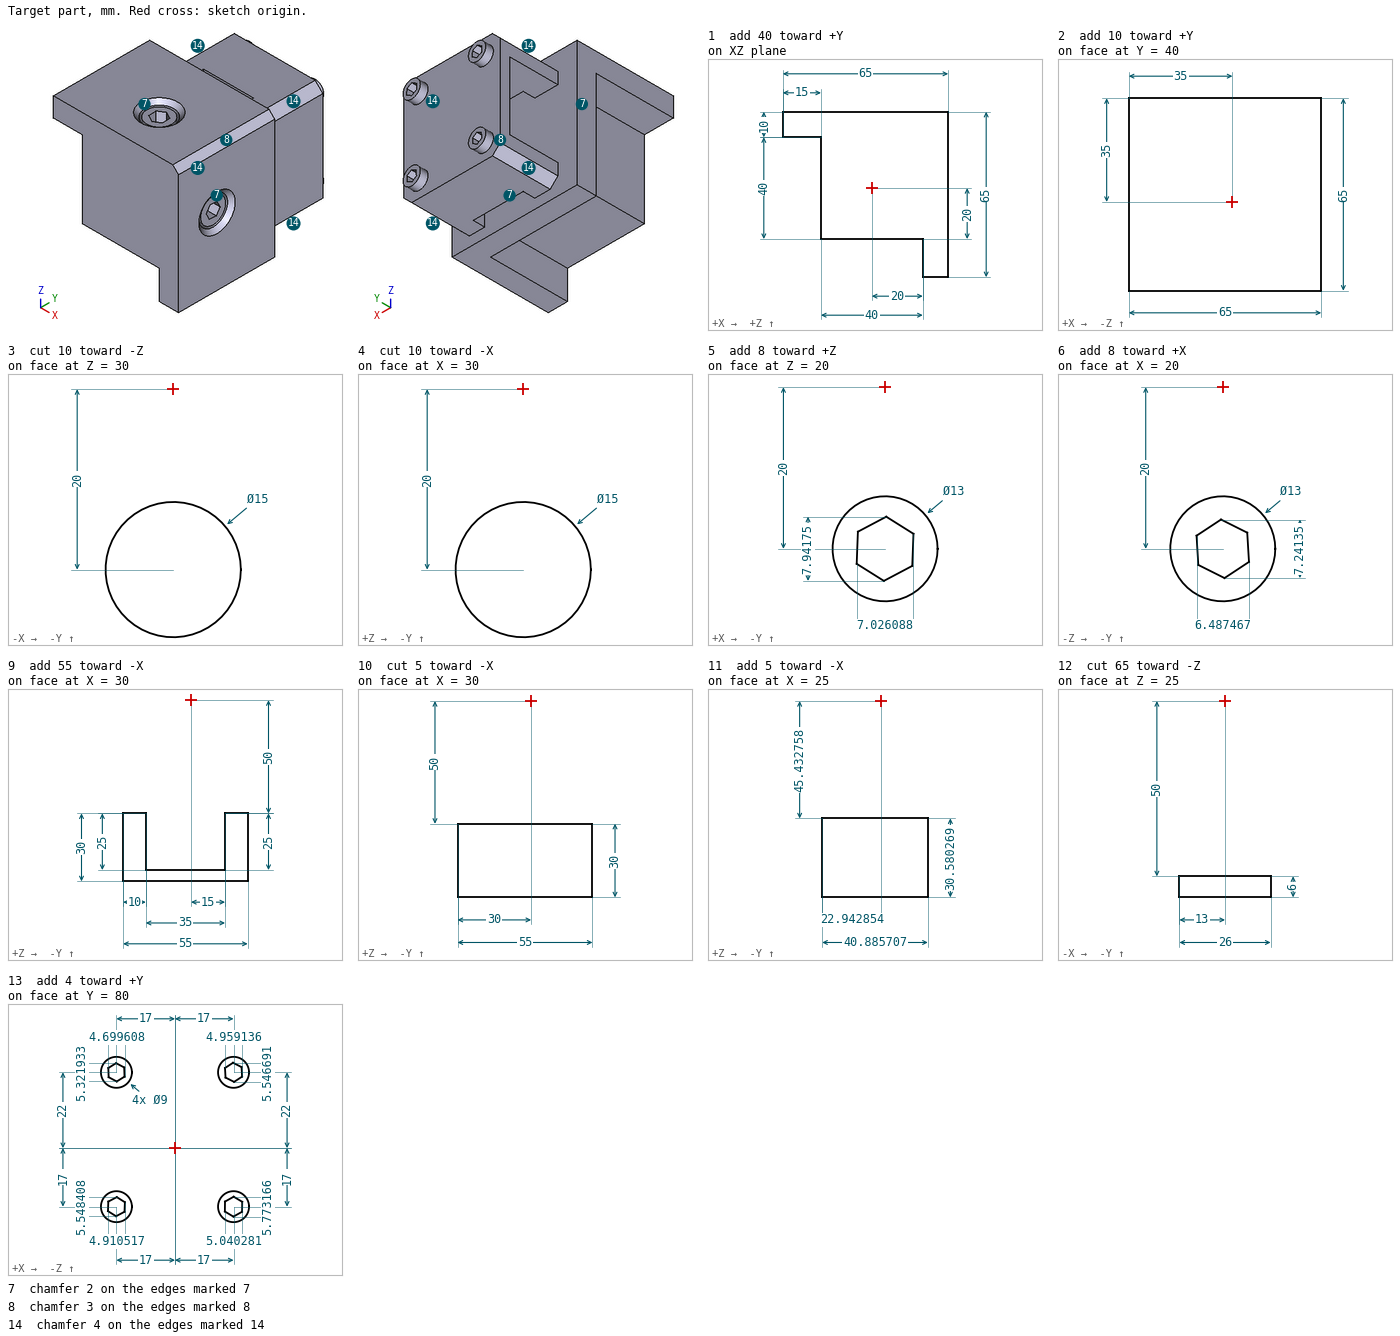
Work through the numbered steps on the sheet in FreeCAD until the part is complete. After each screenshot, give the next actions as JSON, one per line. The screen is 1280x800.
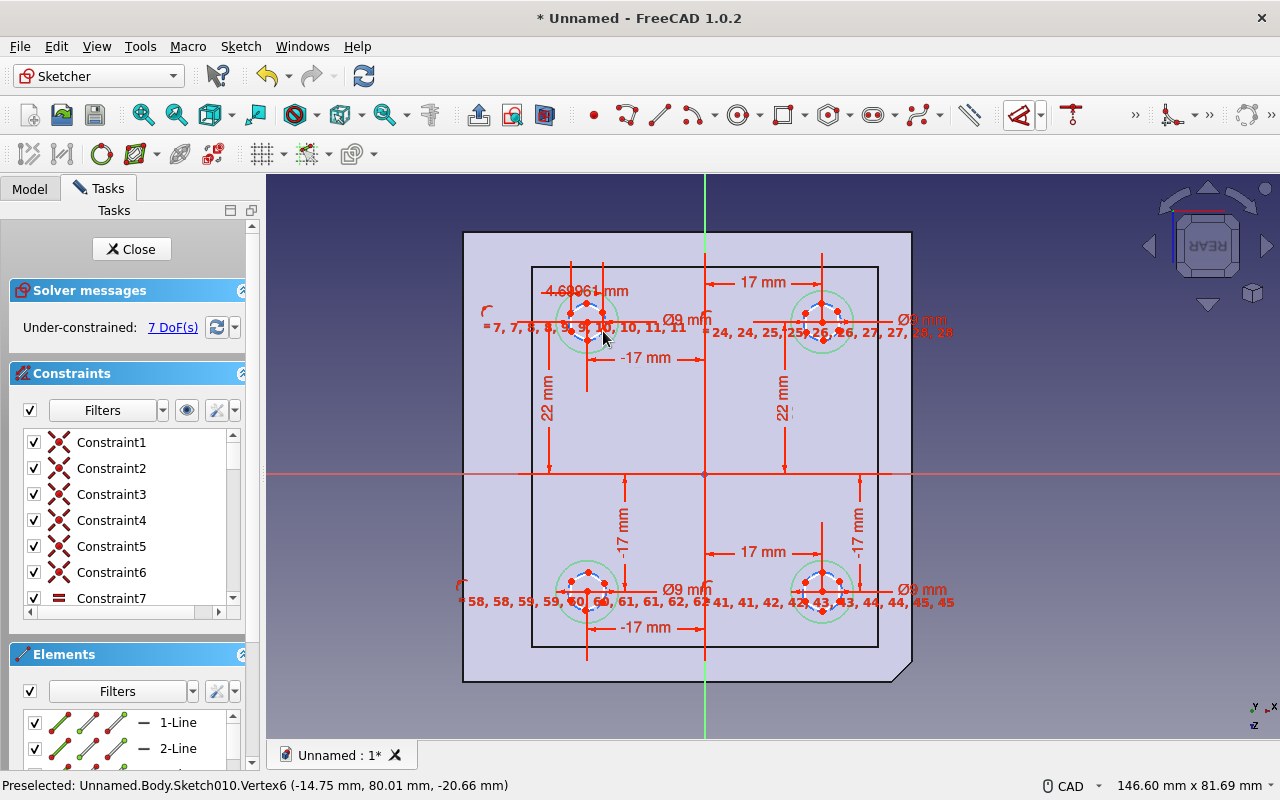
{"action": "left_click", "coordinate": [588, 341]}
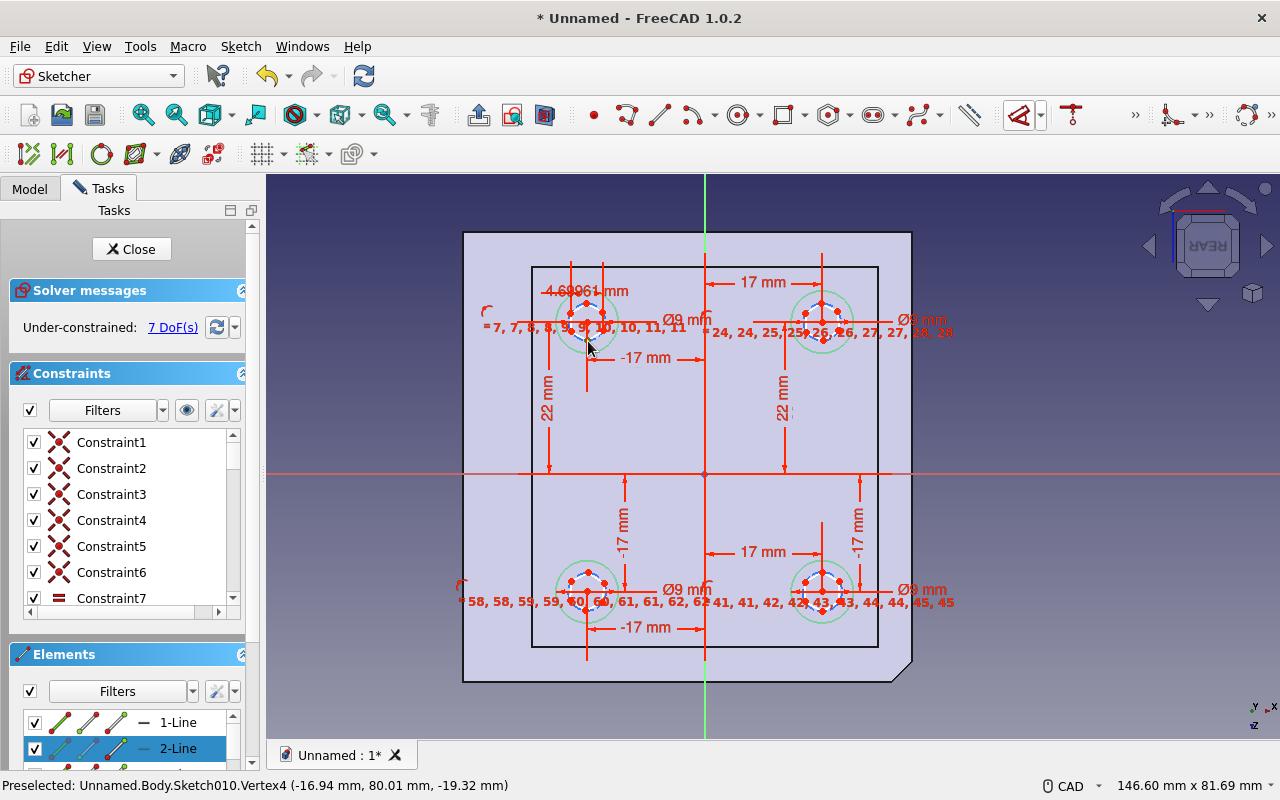
{"action": "left_click", "coordinate": [587, 304]}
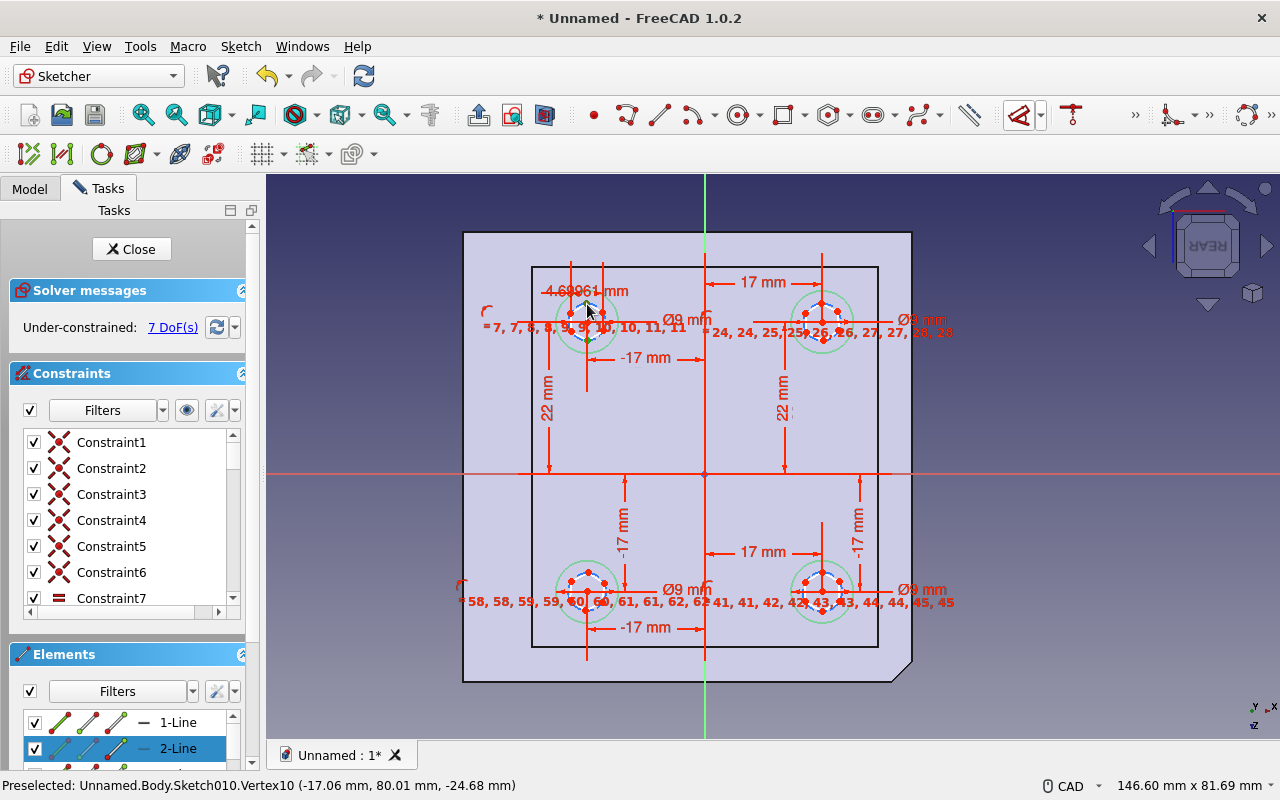
{"action": "key", "text": "i"}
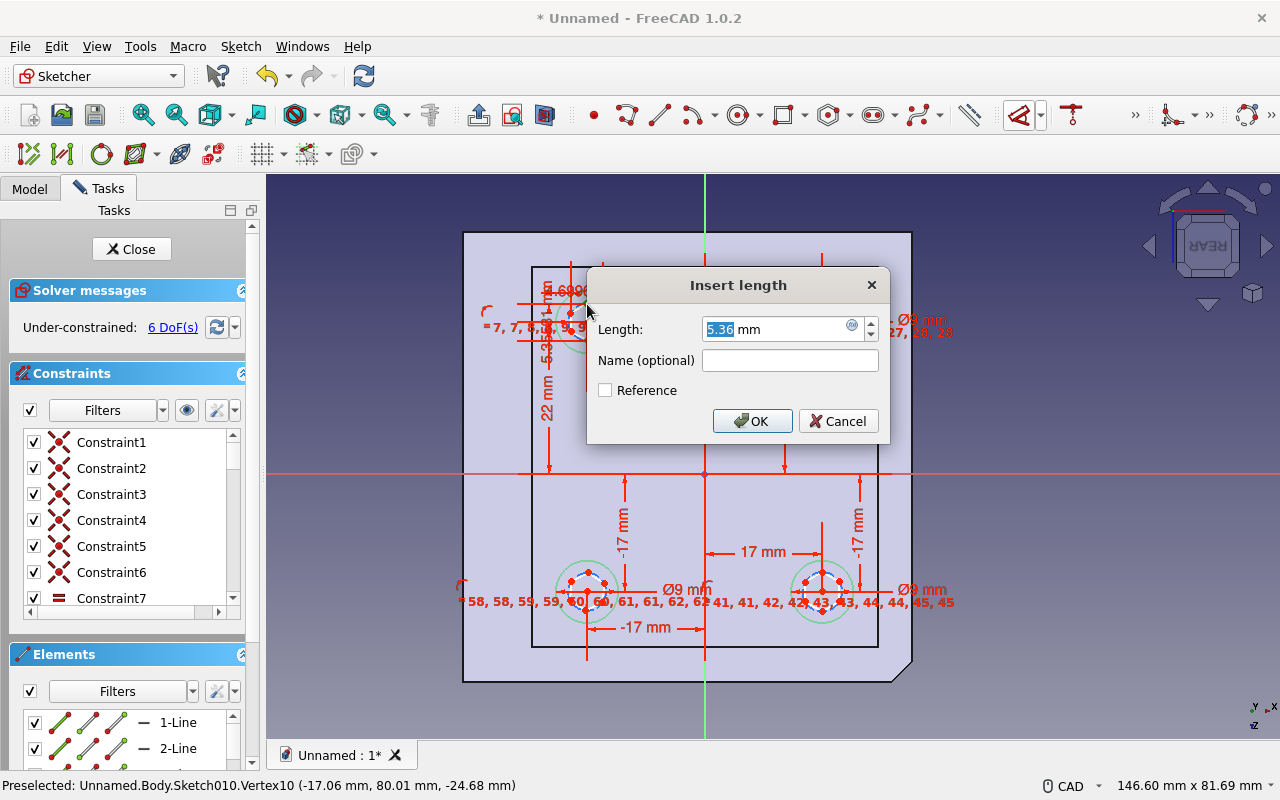
{"action": "type", "text": "5.321933"}
{"action": "key", "text": "Return"}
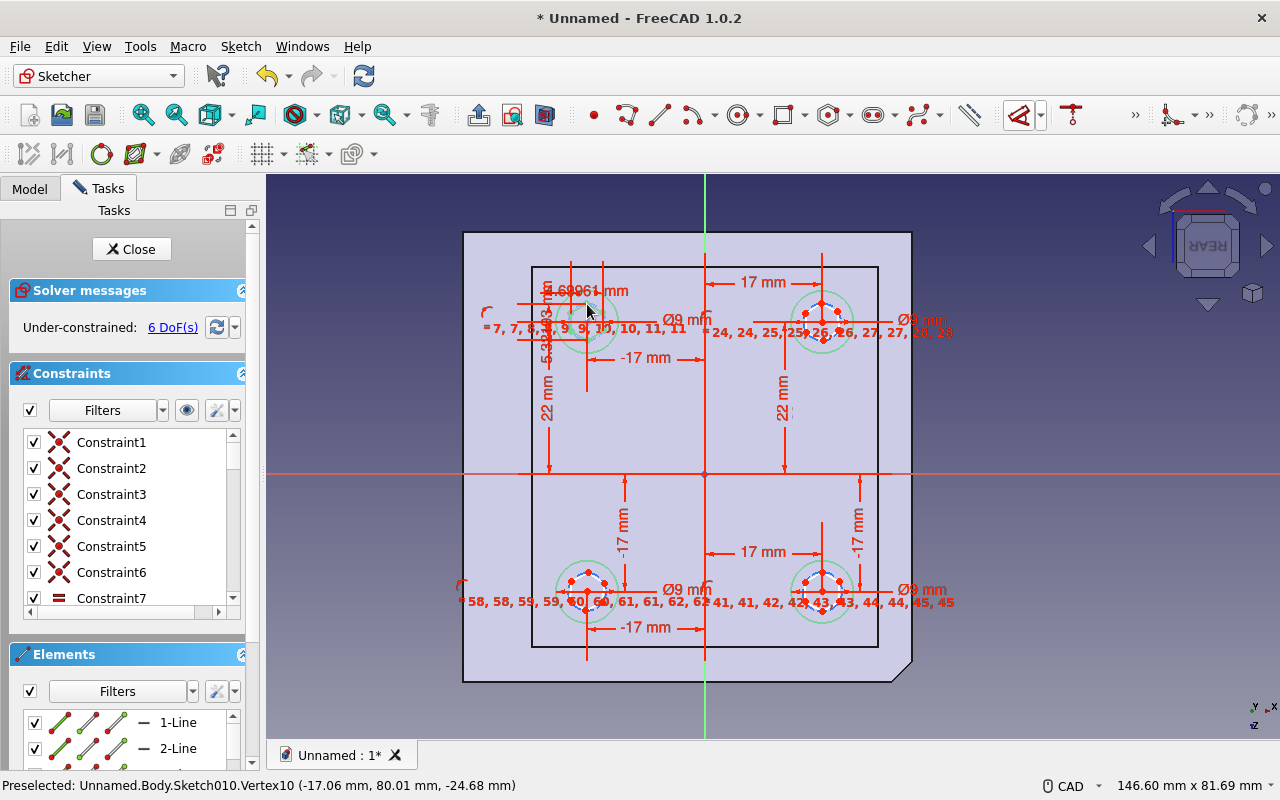
{"action": "left_click", "coordinate": [806, 314]}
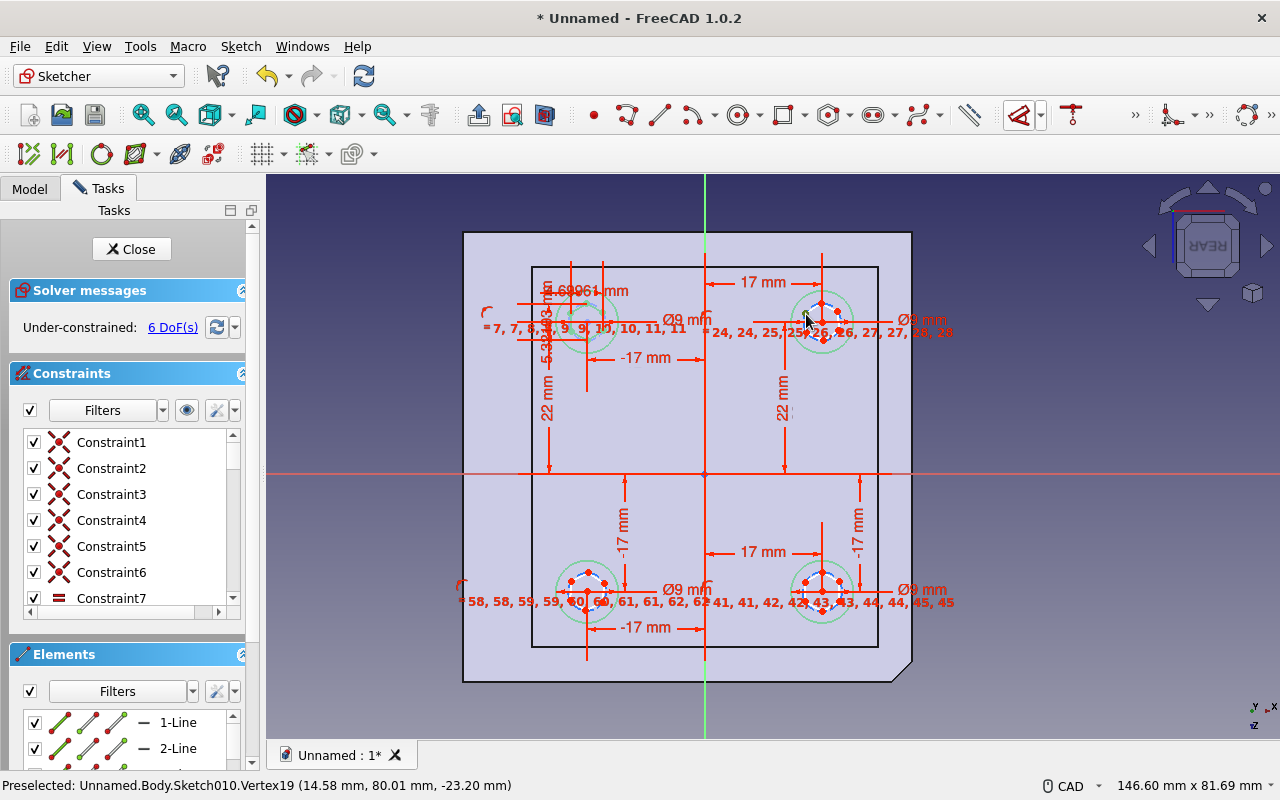
{"action": "left_click", "coordinate": [839, 330]}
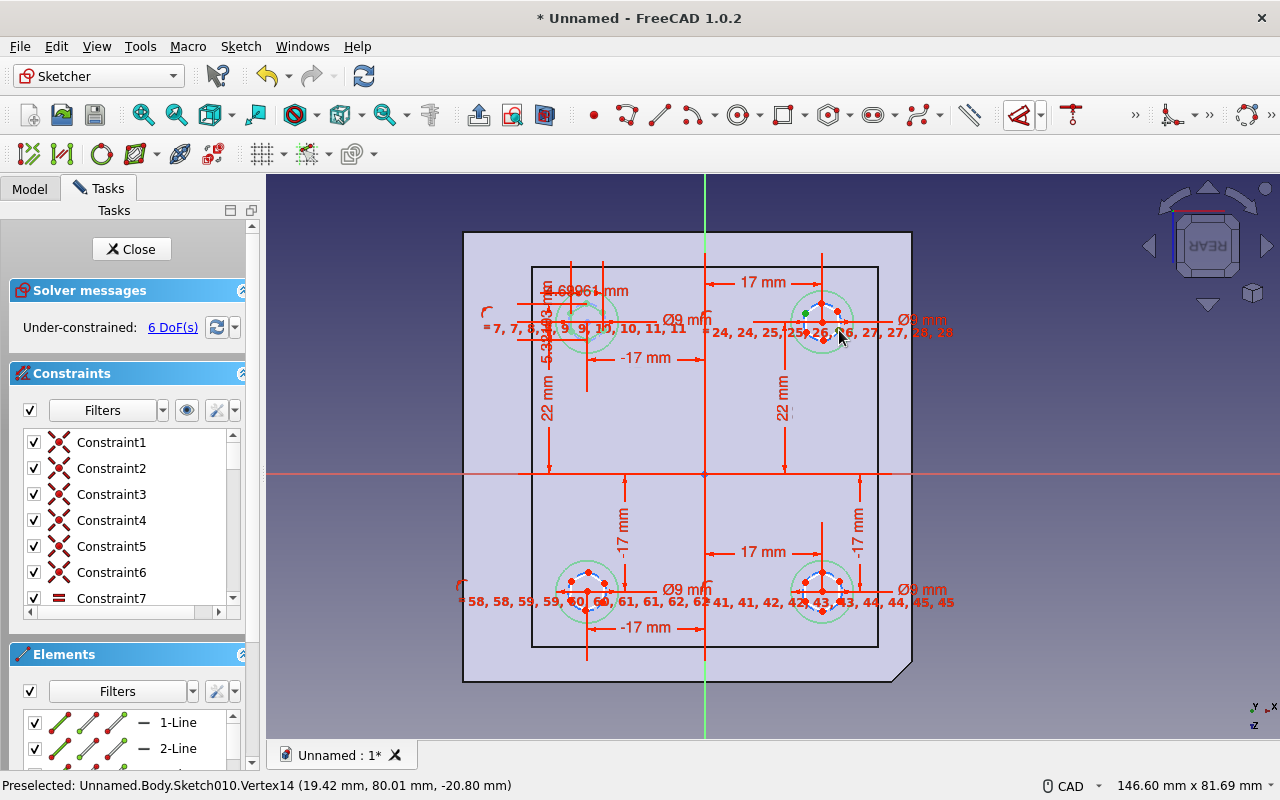
{"action": "left_click", "coordinate": [1040, 116]}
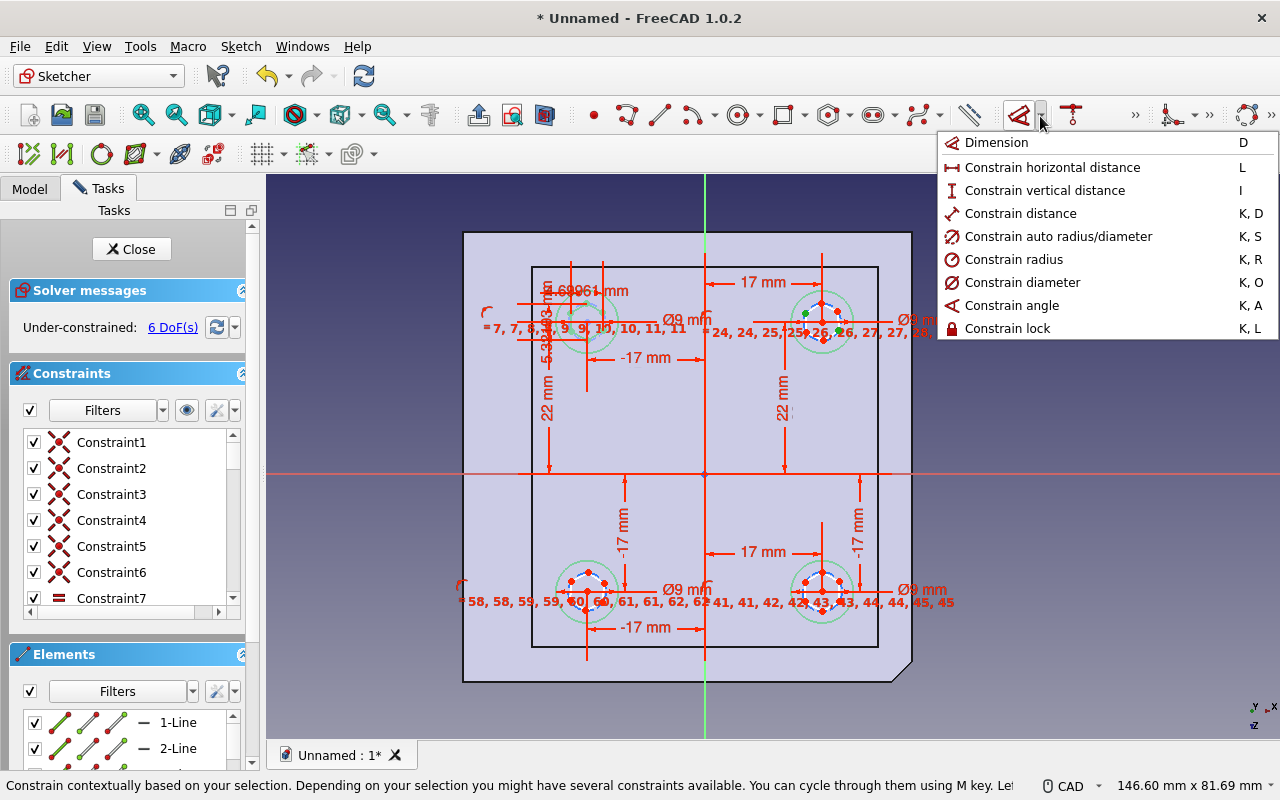
{"action": "left_click", "coordinate": [1108, 168]}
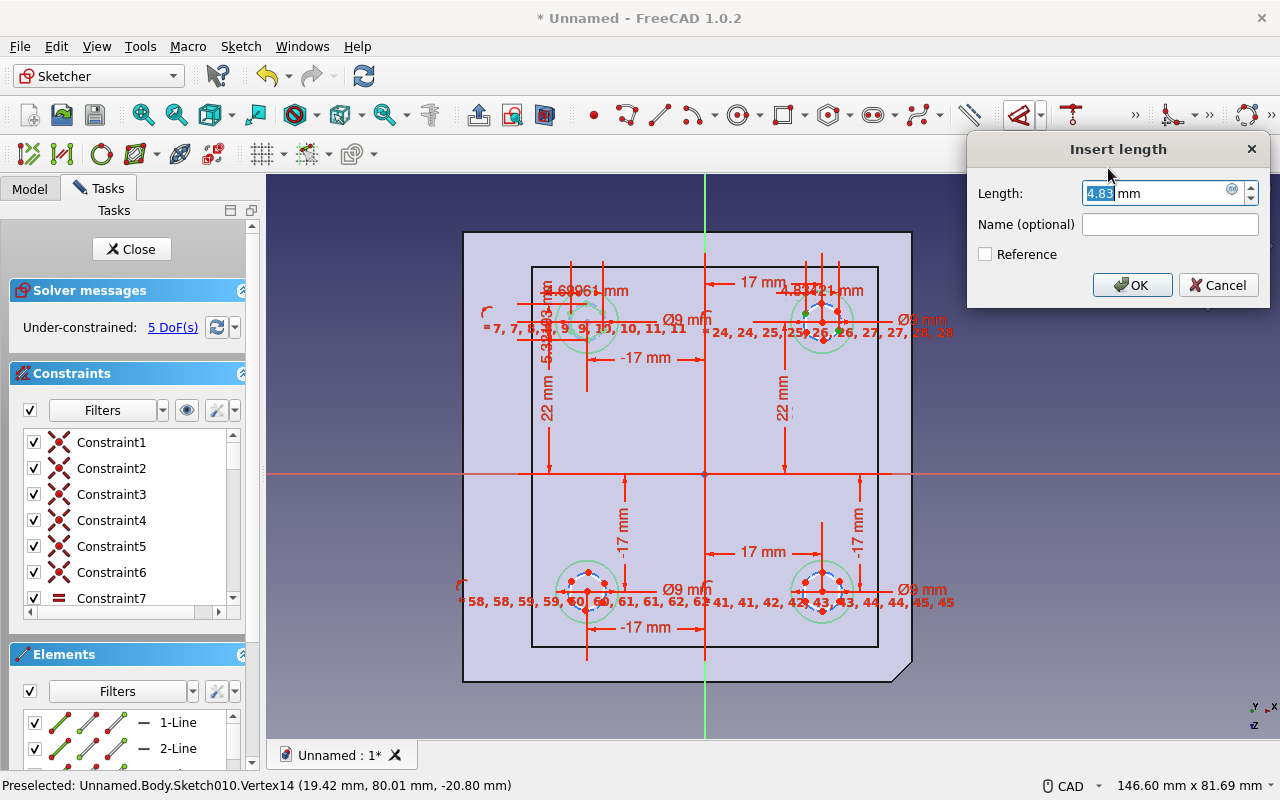
{"action": "type", "text": "4.959136"}
{"action": "key", "text": "Return"}